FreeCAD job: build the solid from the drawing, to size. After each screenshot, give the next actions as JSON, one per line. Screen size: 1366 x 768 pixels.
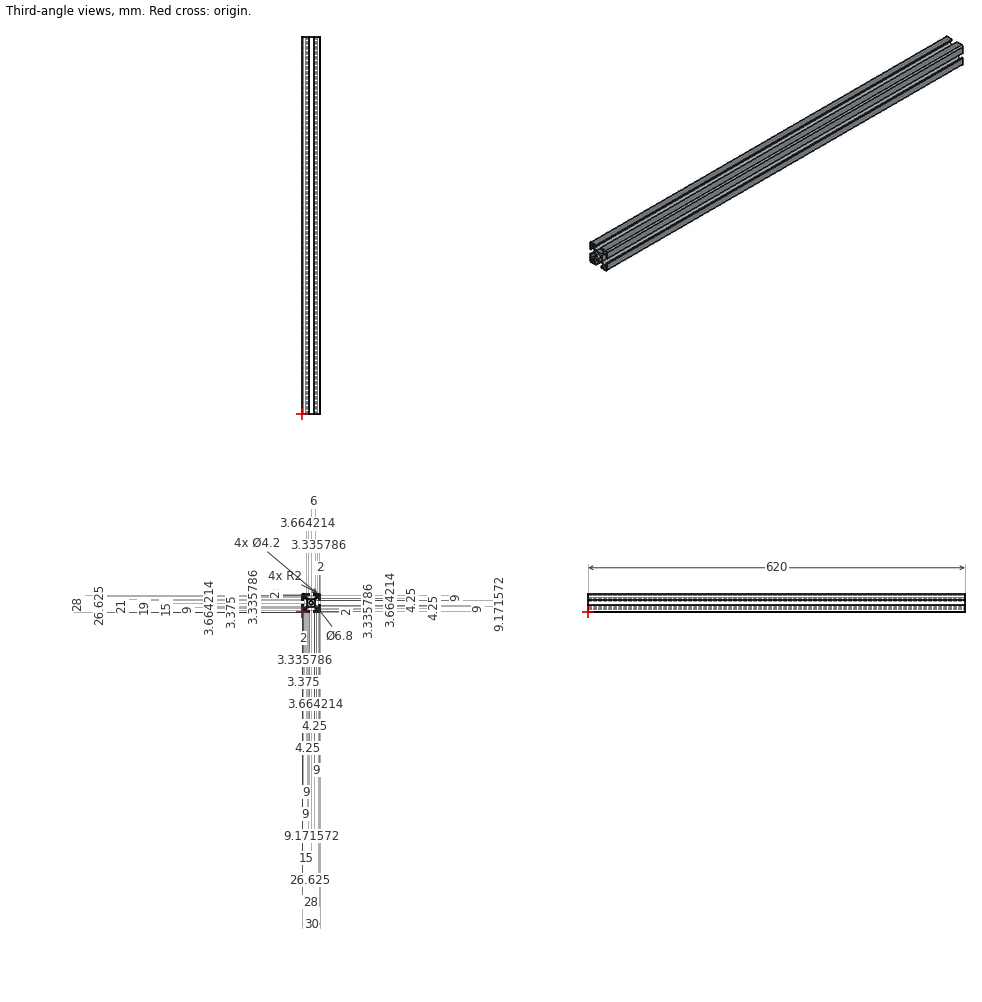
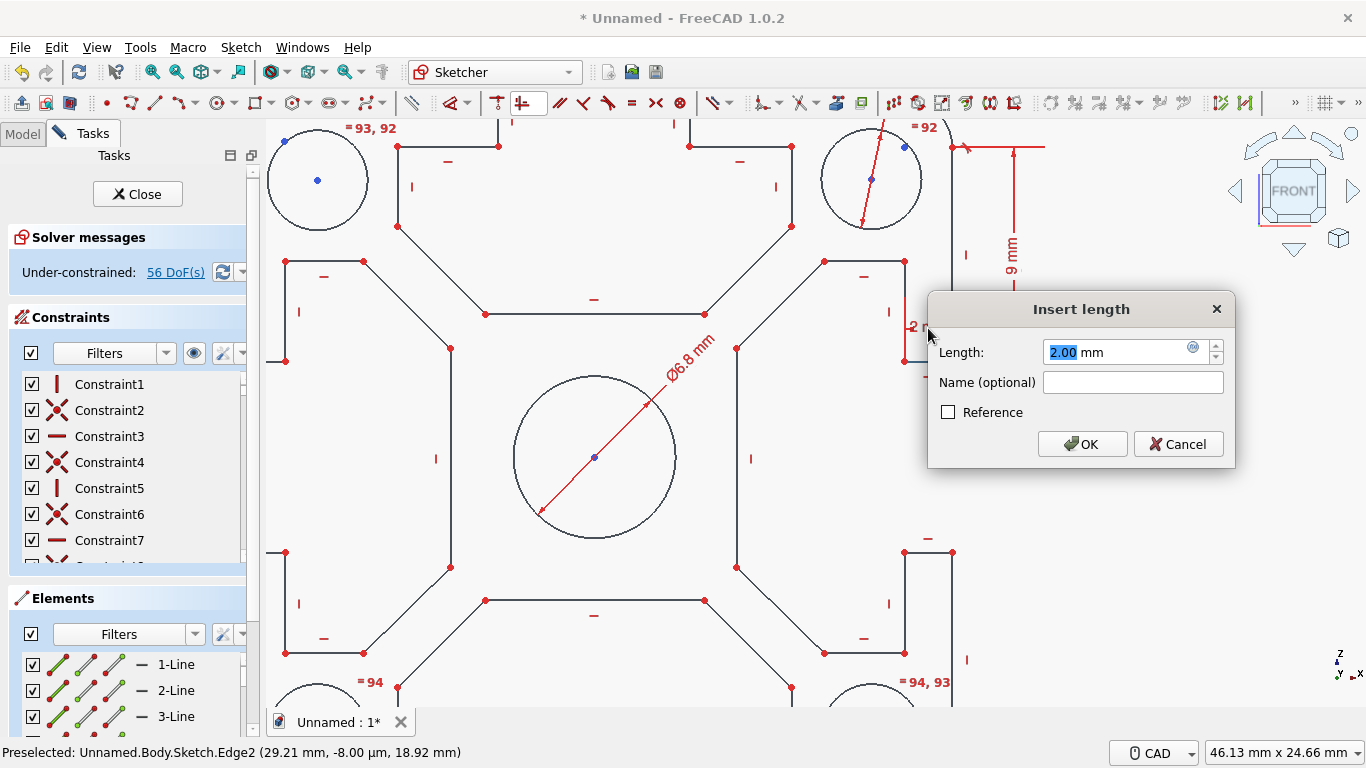
{"action": "type", "text": "2"}
{"action": "key", "text": "Return"}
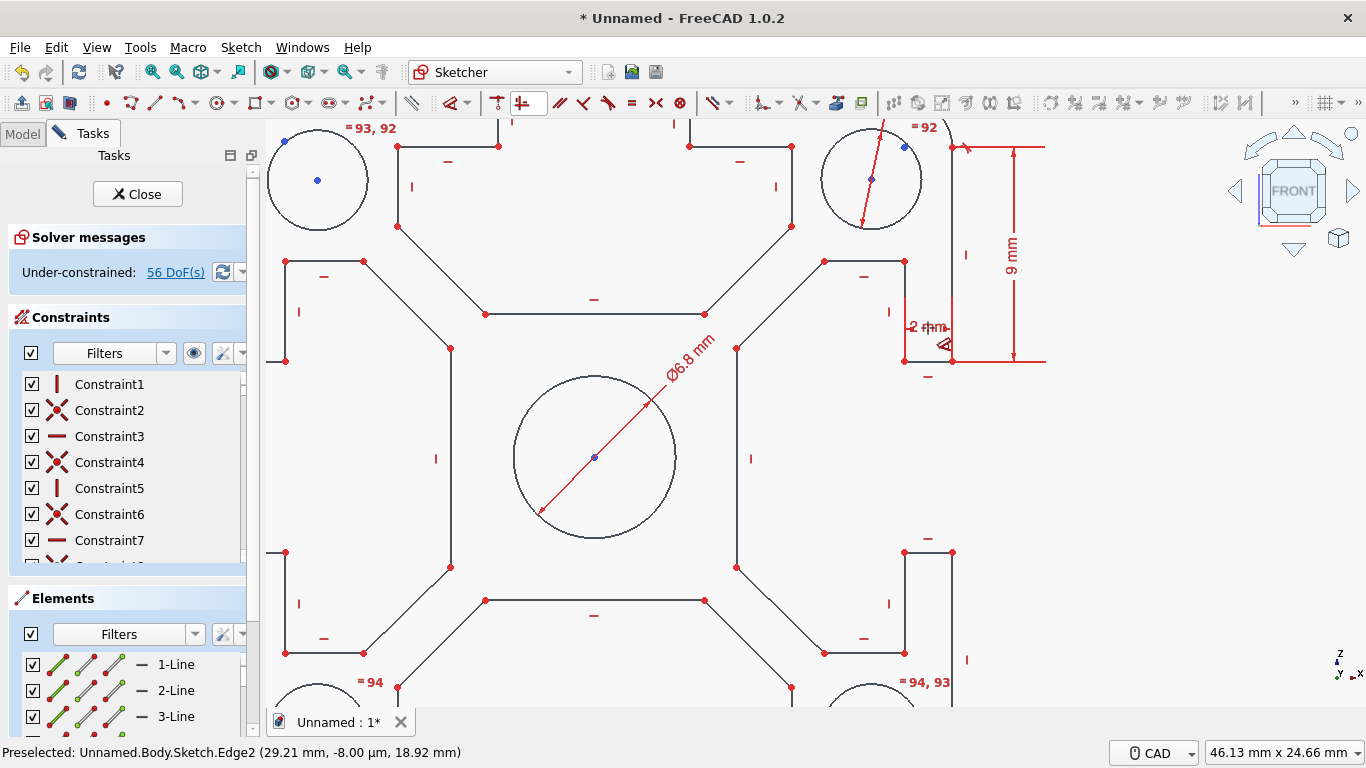
{"action": "left_click", "coordinate": [919, 553]}
{"action": "left_click", "coordinate": [929, 587]}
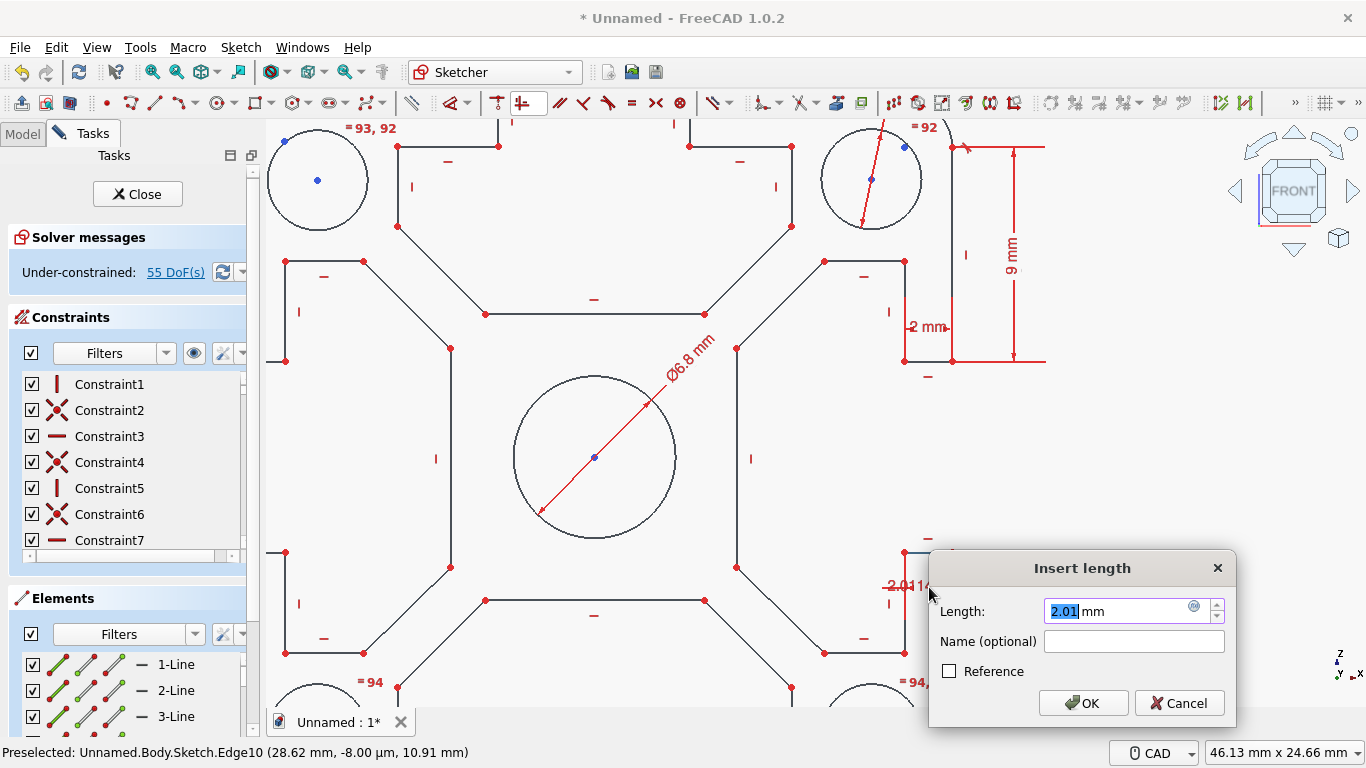
{"action": "type", "text": "2"}
{"action": "key", "text": "Return"}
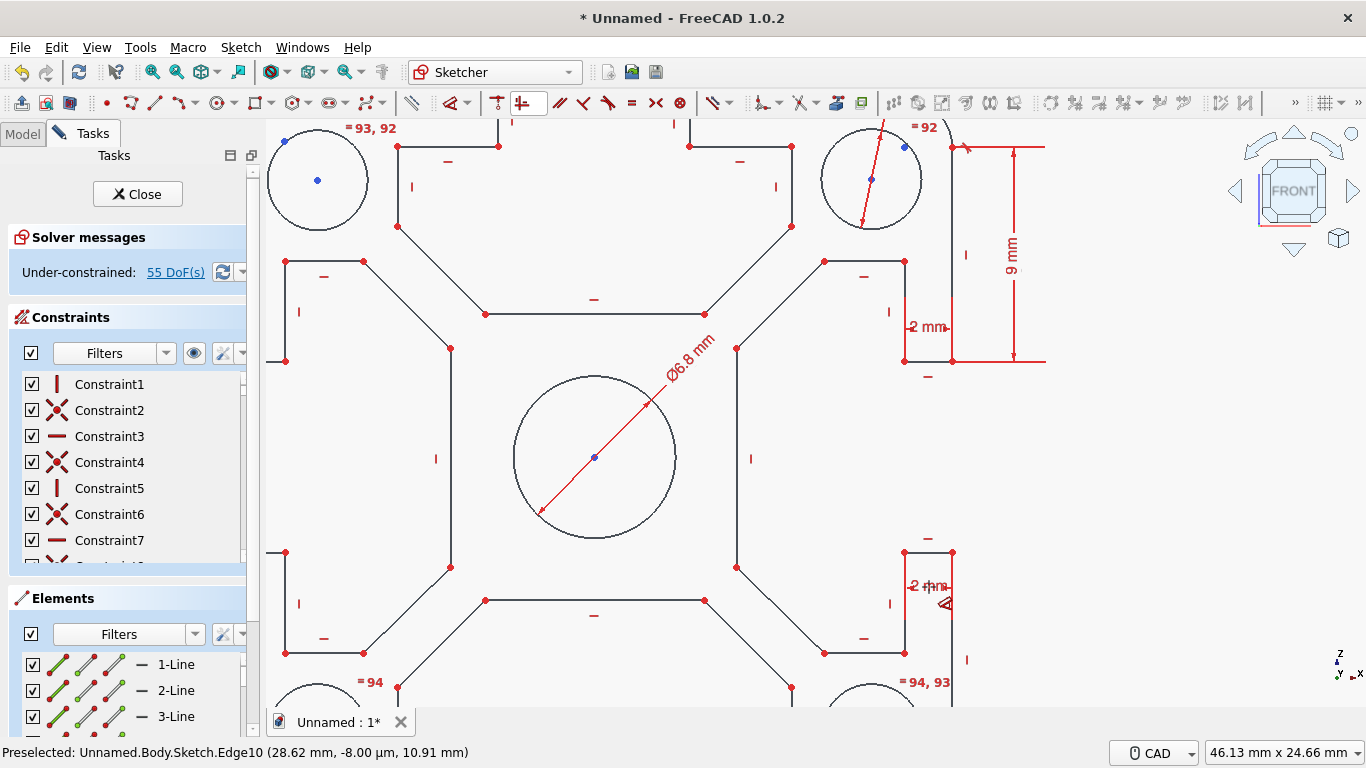
{"action": "left_click", "coordinate": [952, 617]}
{"action": "left_click", "coordinate": [986, 616]}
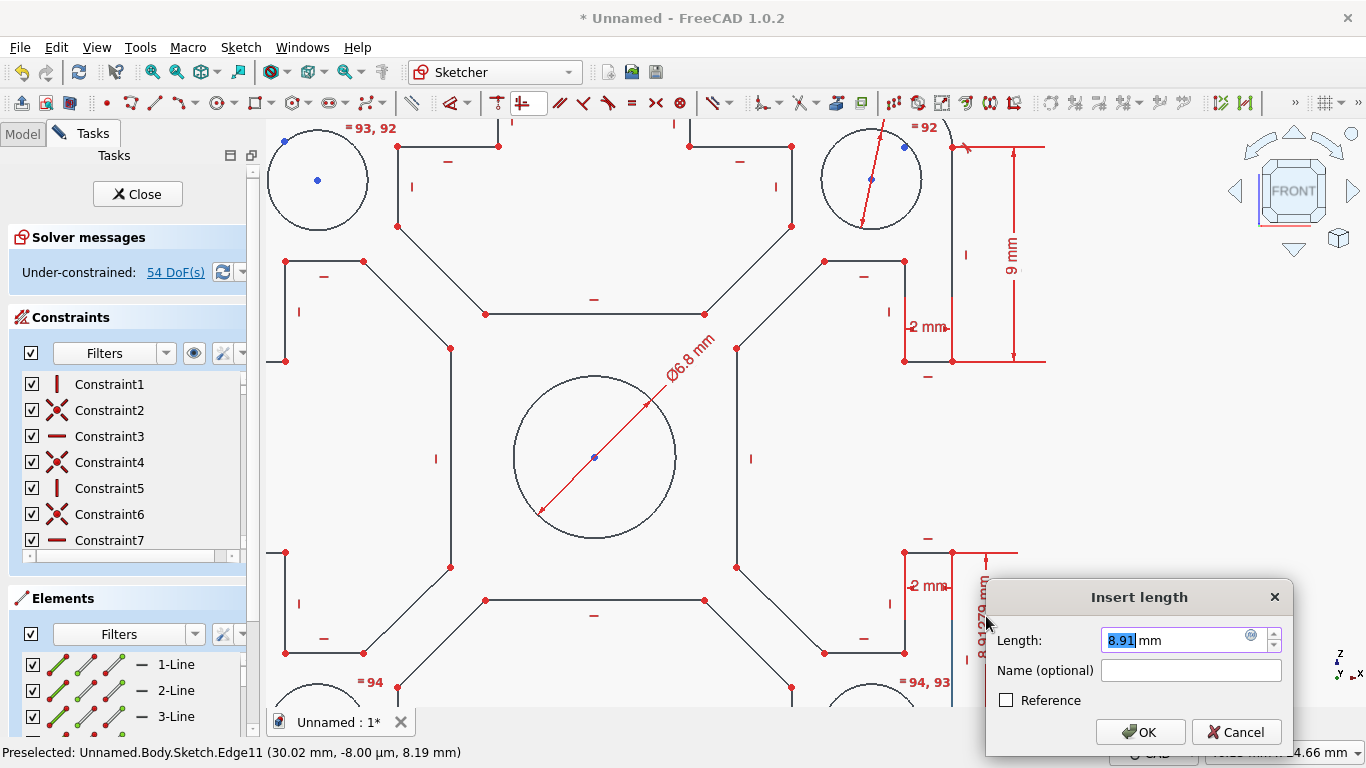
{"action": "type", "text": "9"}
{"action": "key", "text": "Return"}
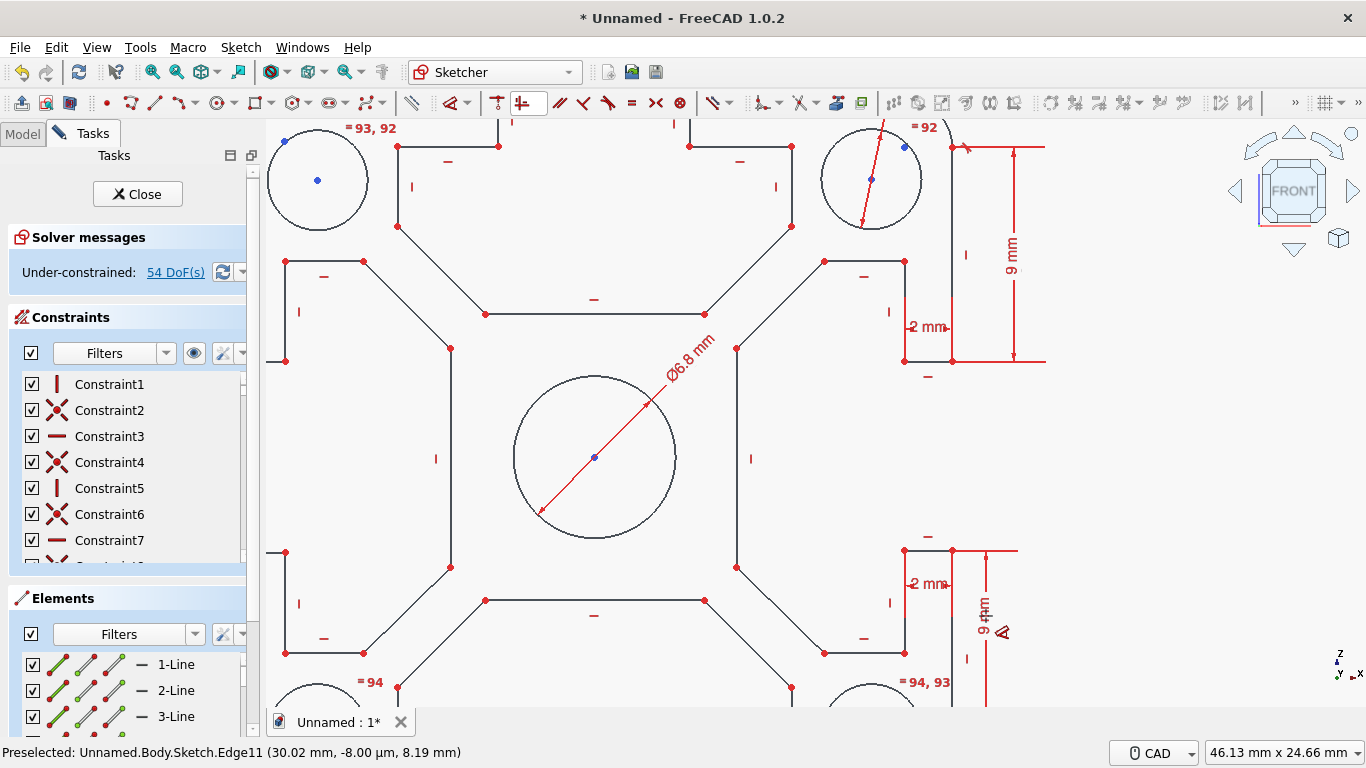
{"action": "scroll", "coordinate": [934, 361], "scroll_direction": "down", "scroll_amount": 3}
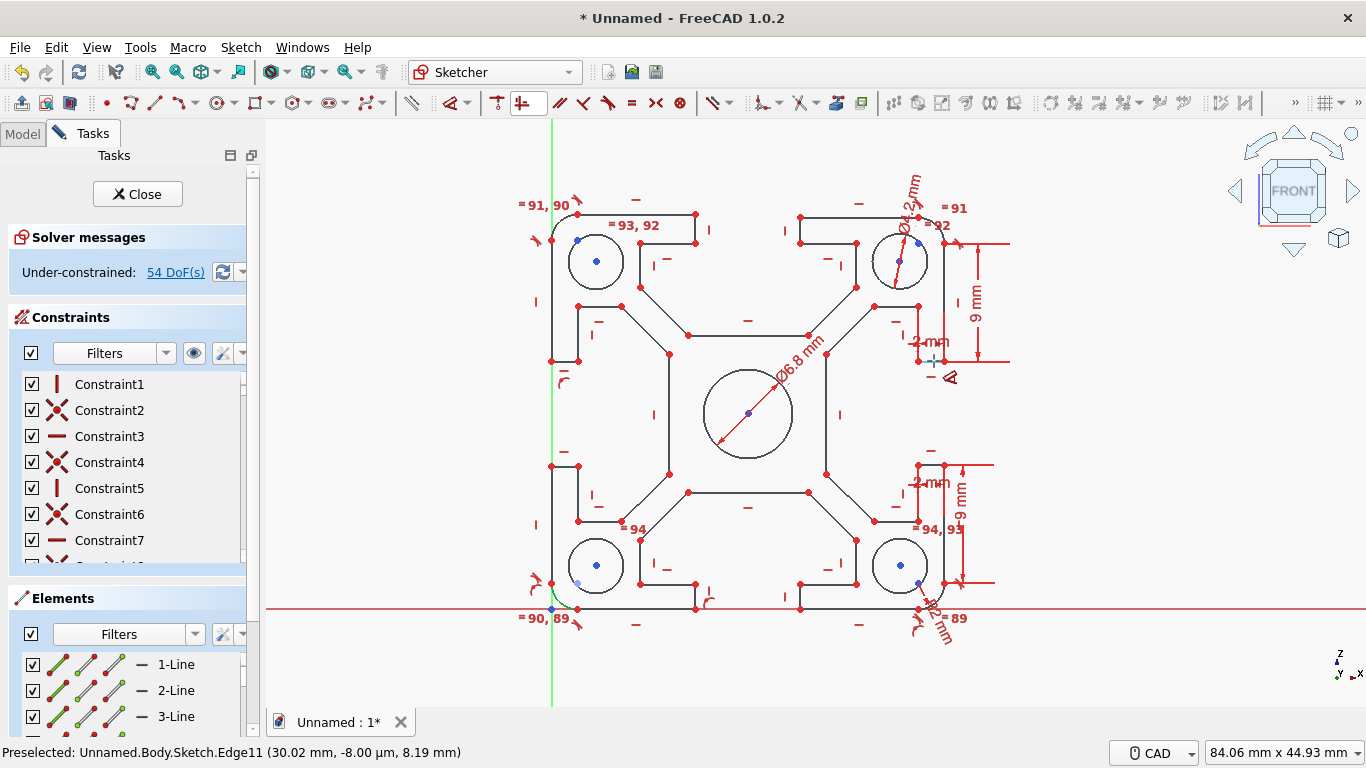
{"action": "left_click", "coordinate": [883, 609]}
{"action": "left_click", "coordinate": [859, 643]}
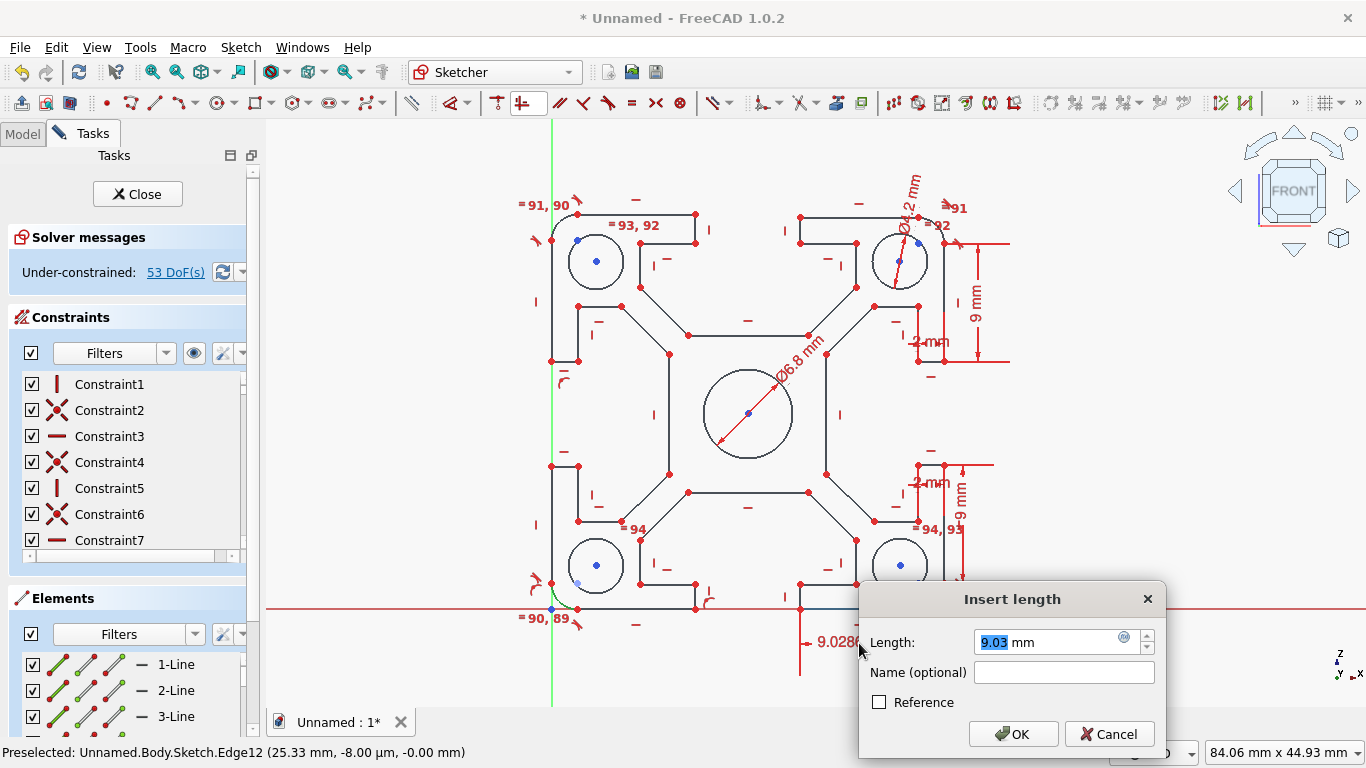
{"action": "type", "text": "9"}
{"action": "key", "text": "Return"}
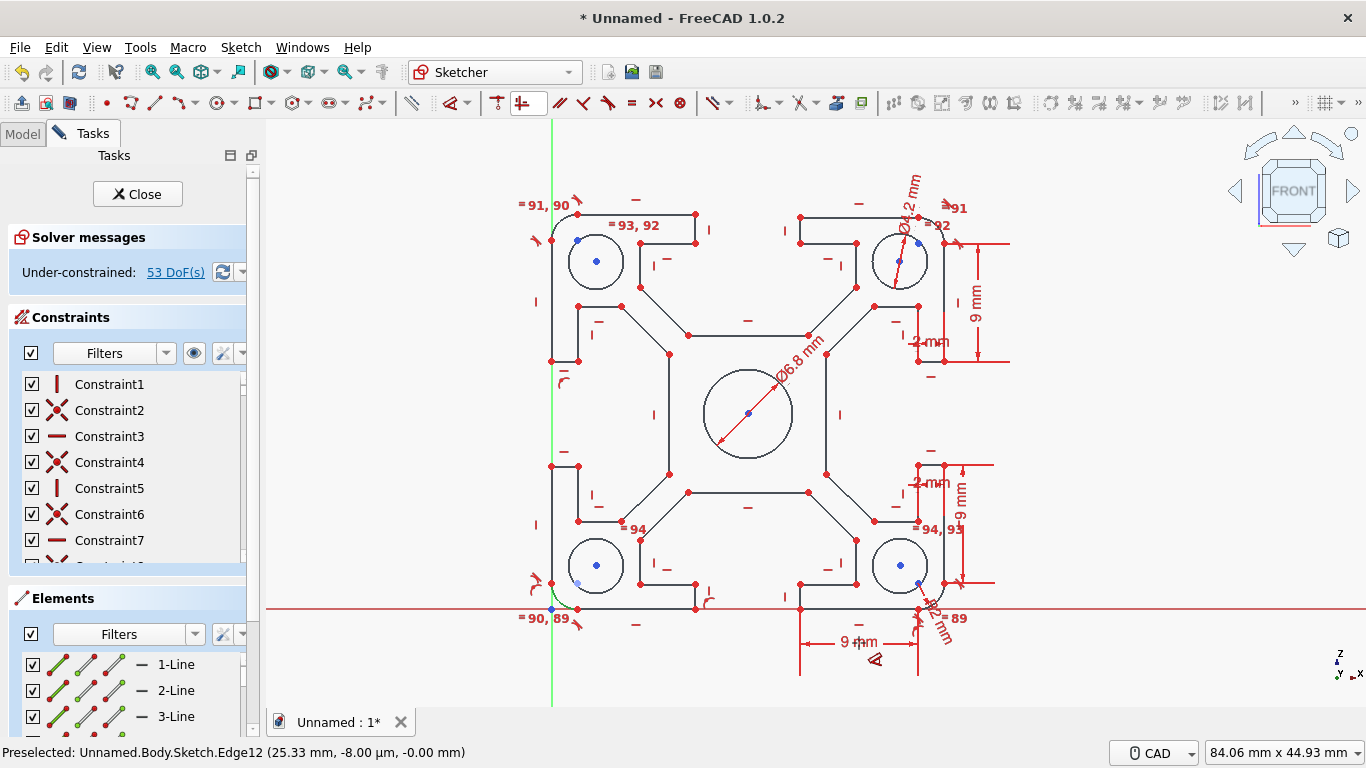
{"action": "scroll", "coordinate": [800, 599], "scroll_direction": "up", "scroll_amount": 3}